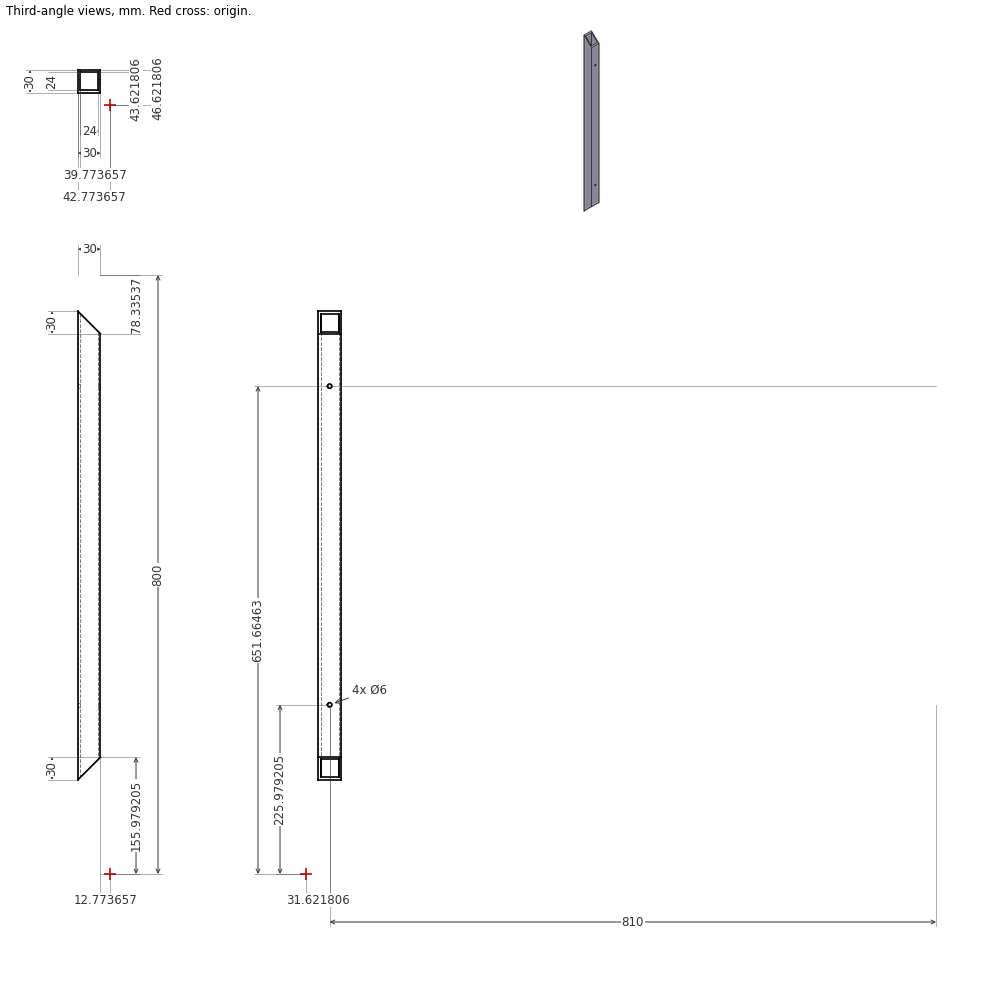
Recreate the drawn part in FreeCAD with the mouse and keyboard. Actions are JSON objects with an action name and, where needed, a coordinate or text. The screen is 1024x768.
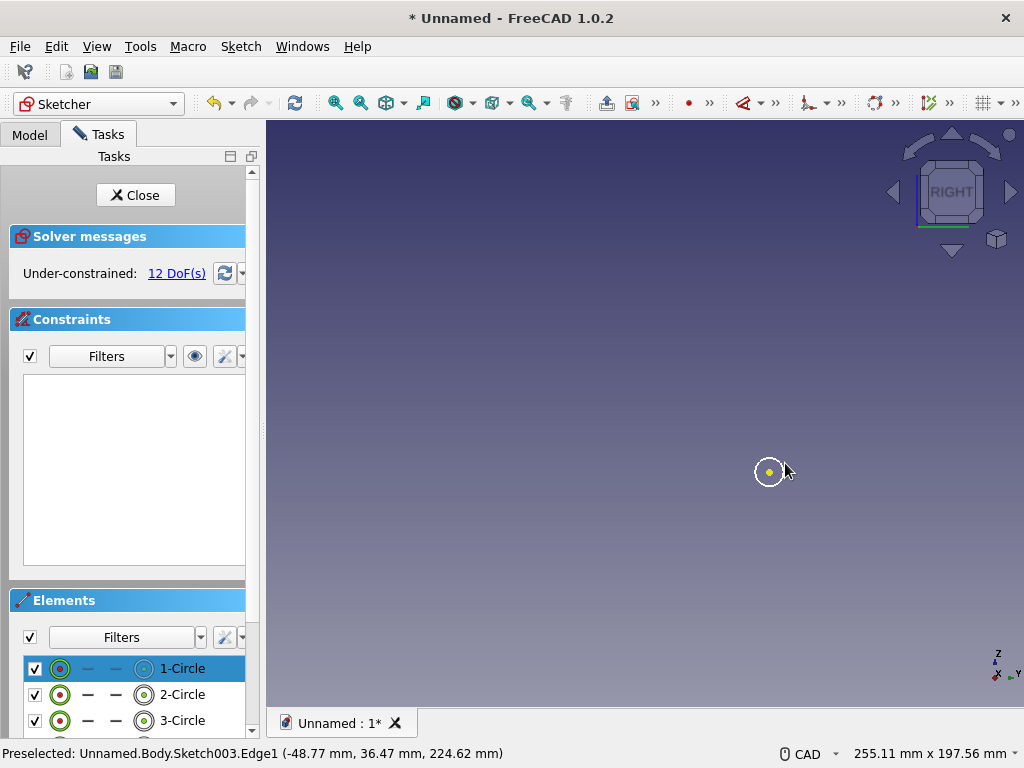
{"action": "left_click", "coordinate": [779, 462]}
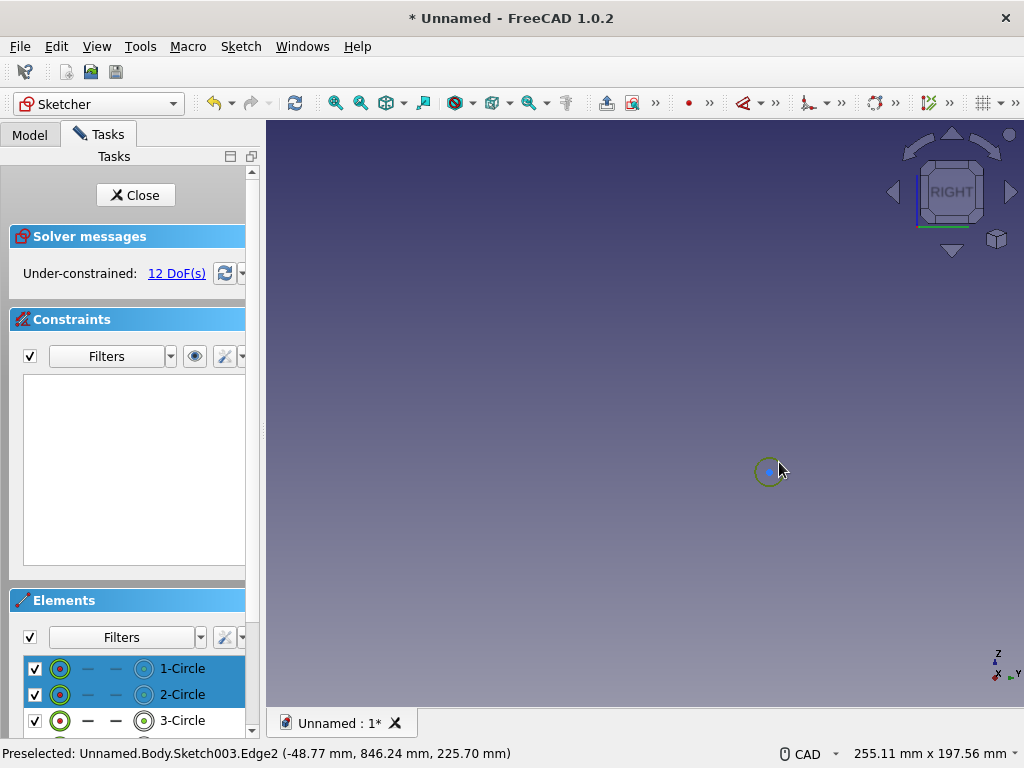
{"action": "scroll", "coordinate": [785, 463], "scroll_direction": "down", "scroll_amount": 9}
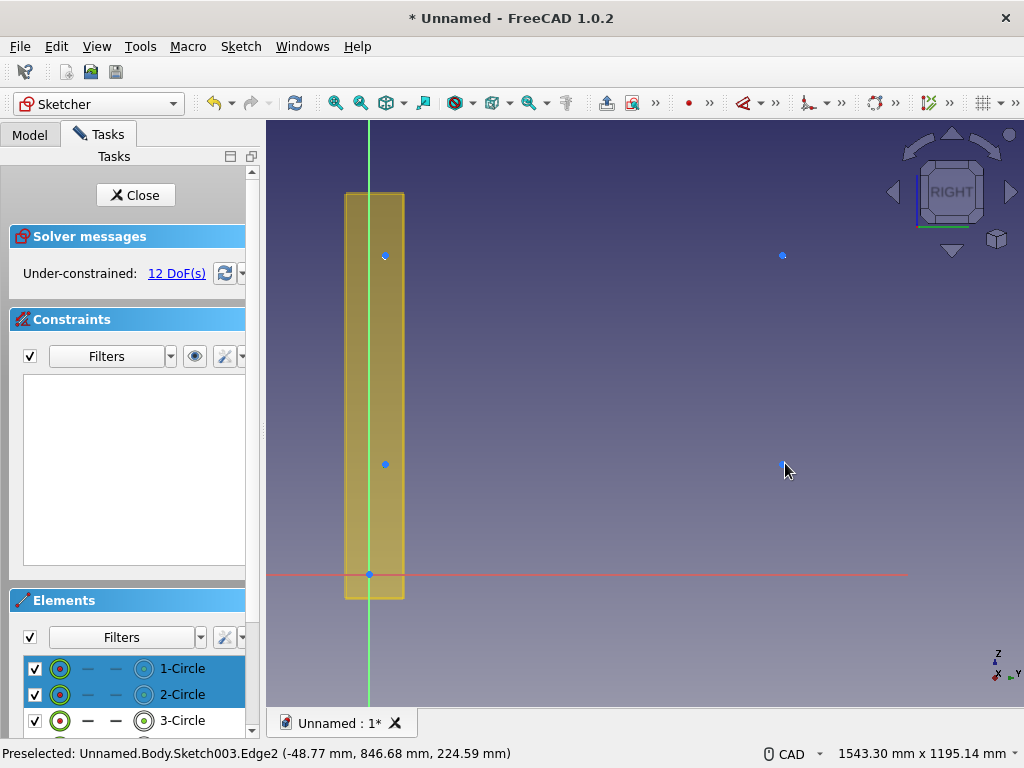
{"action": "scroll", "coordinate": [785, 254], "scroll_direction": "up", "scroll_amount": 9}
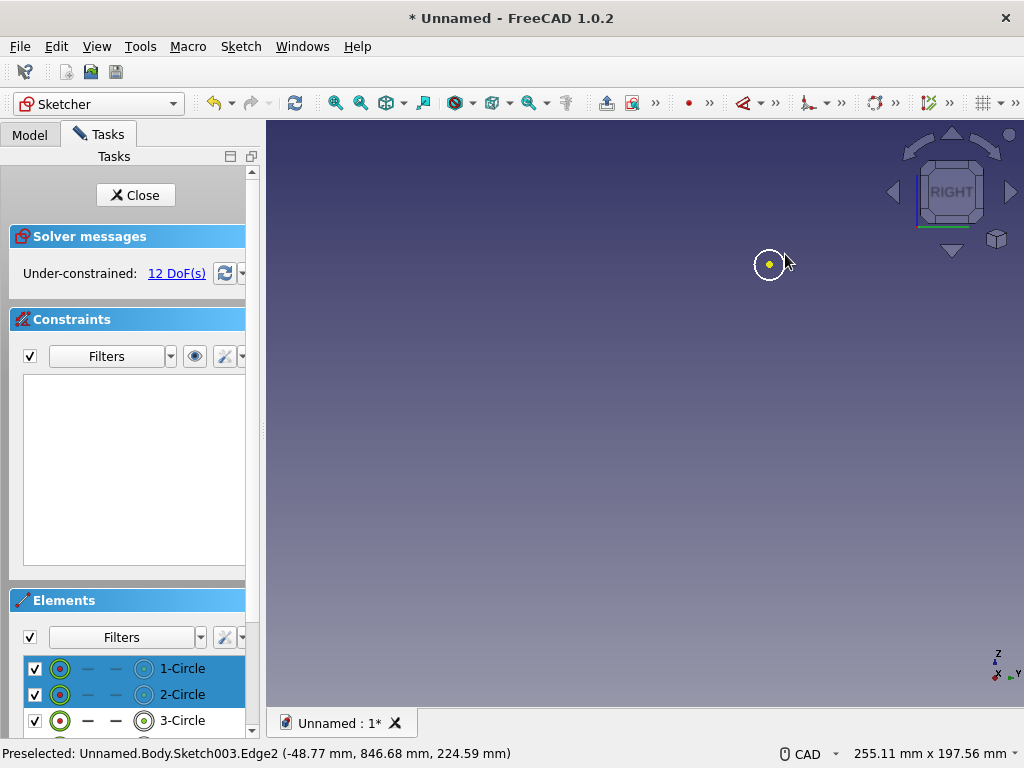
{"action": "left_click", "coordinate": [780, 254]}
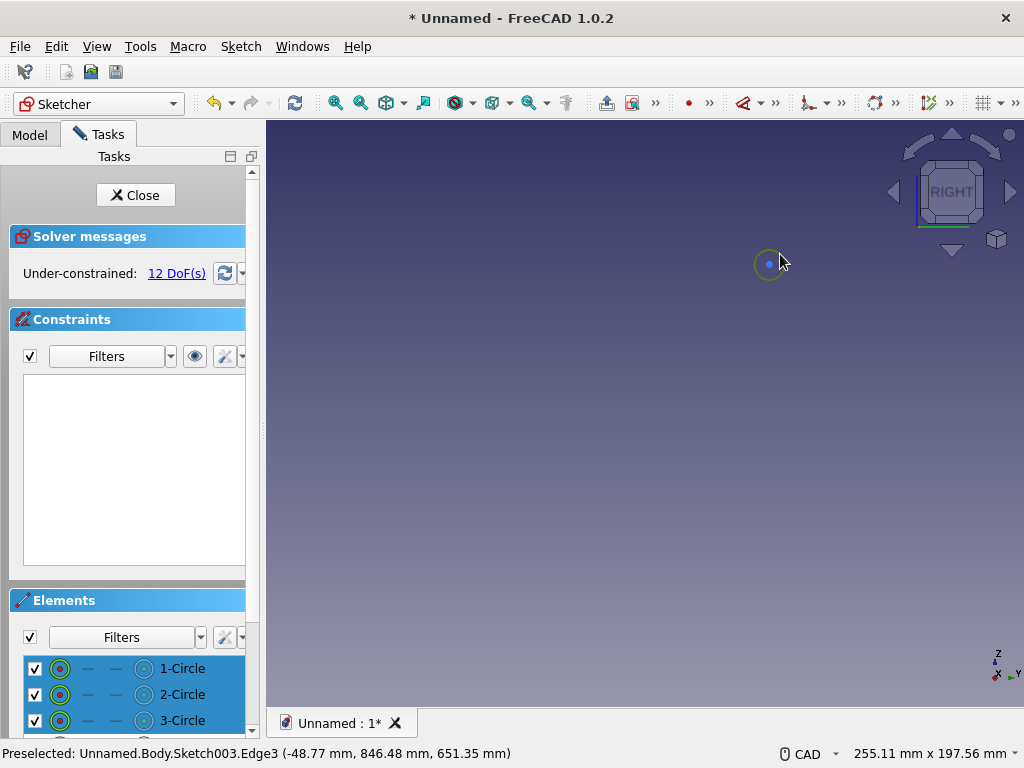
{"action": "scroll", "coordinate": [785, 254], "scroll_direction": "down", "scroll_amount": 9}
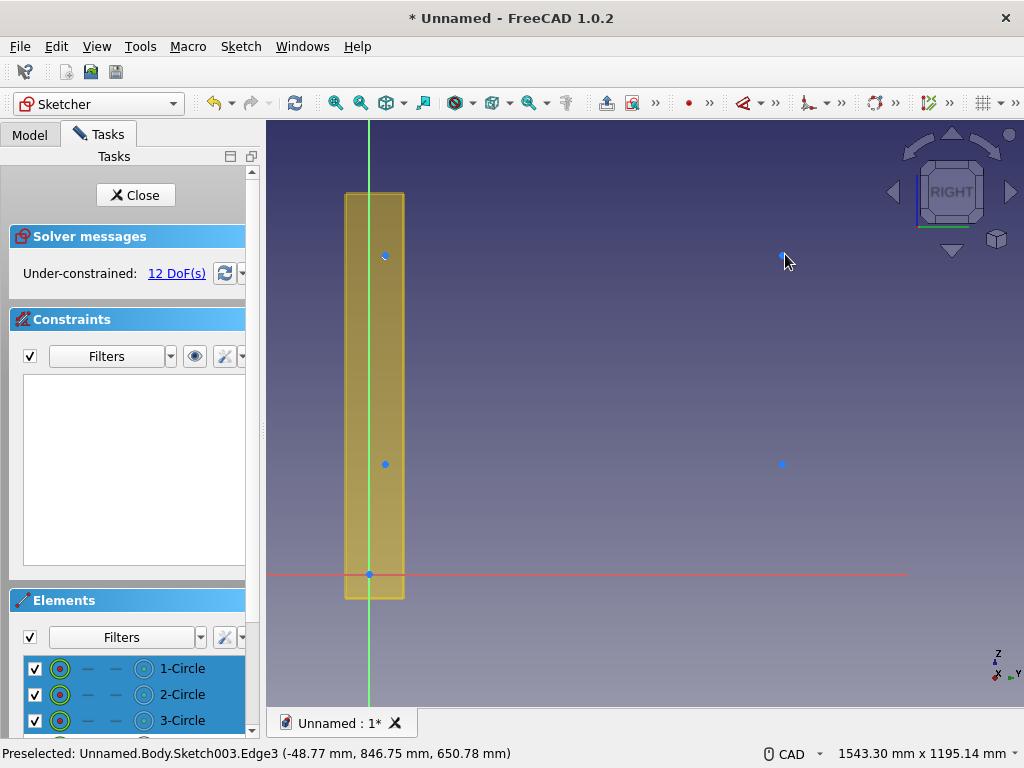
{"action": "scroll", "coordinate": [387, 254], "scroll_direction": "up", "scroll_amount": 9}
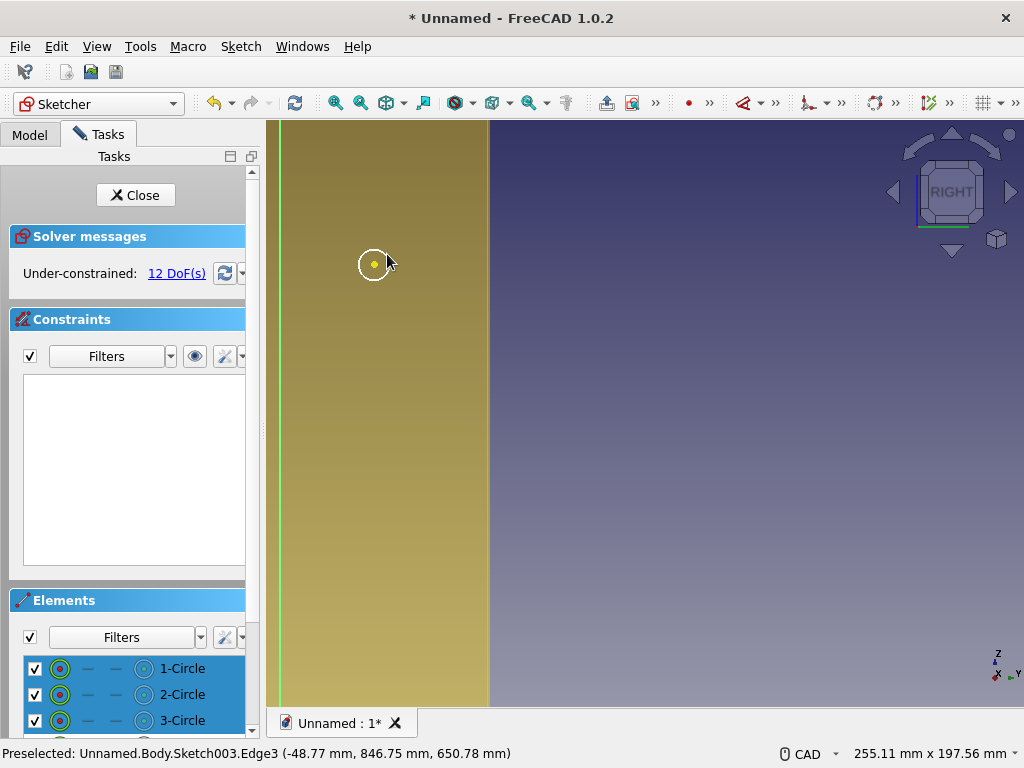
{"action": "left_click", "coordinate": [385, 254]}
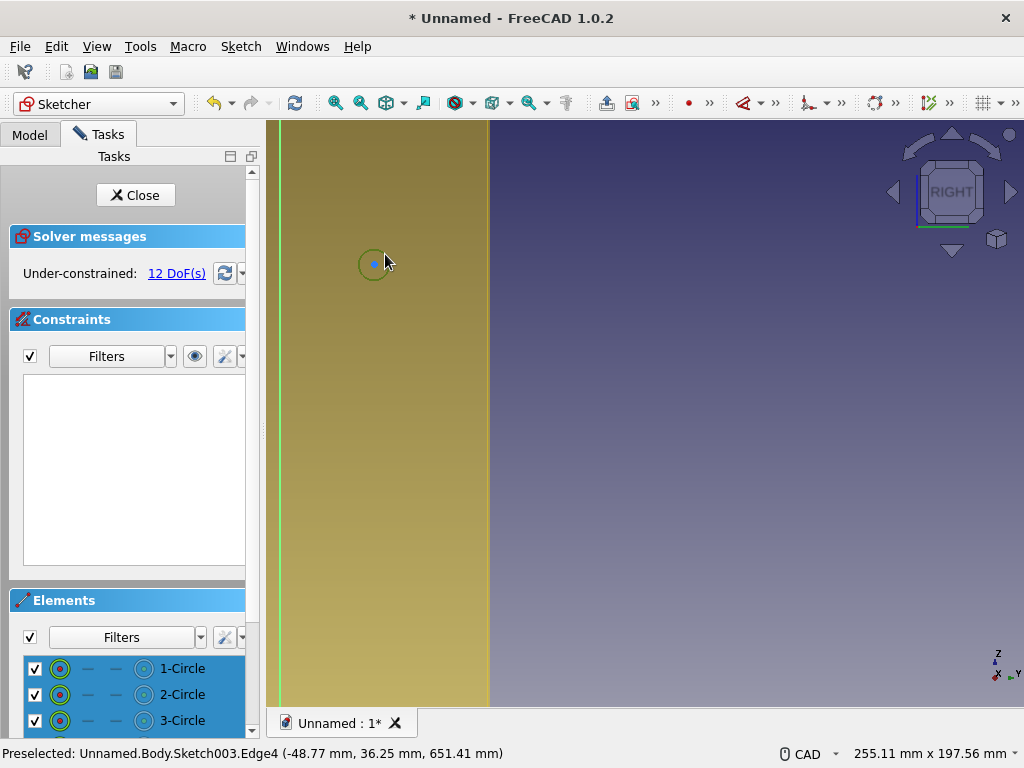
{"action": "key", "text": "e"}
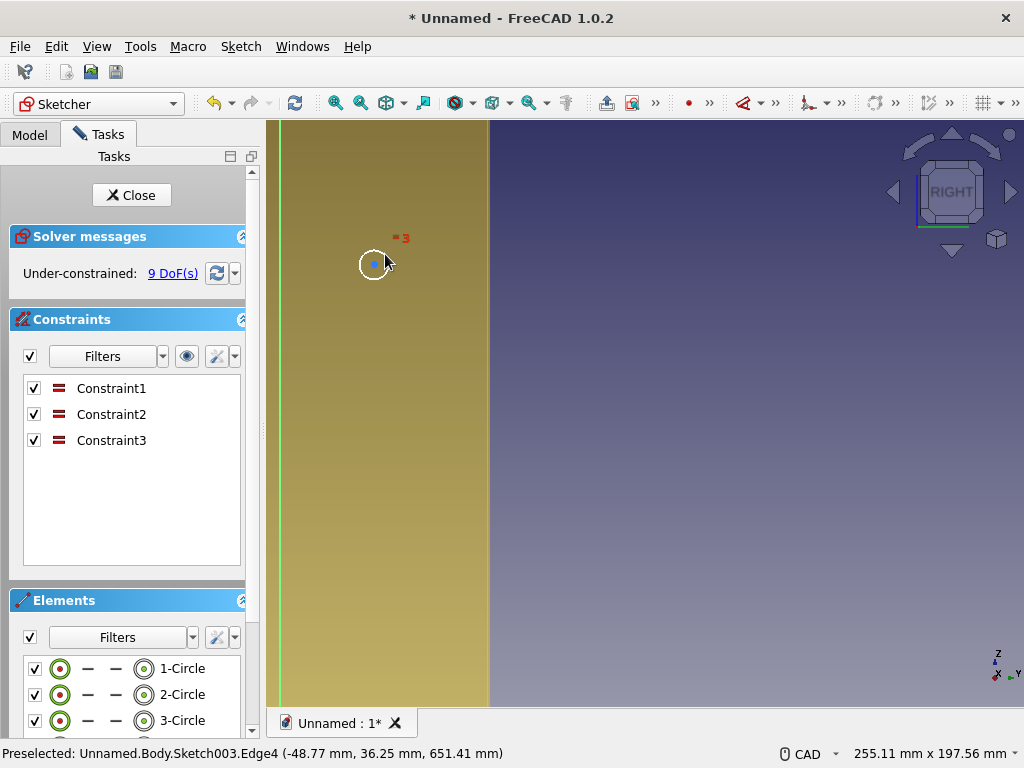
{"action": "scroll", "coordinate": [387, 254], "scroll_direction": "down", "scroll_amount": 9}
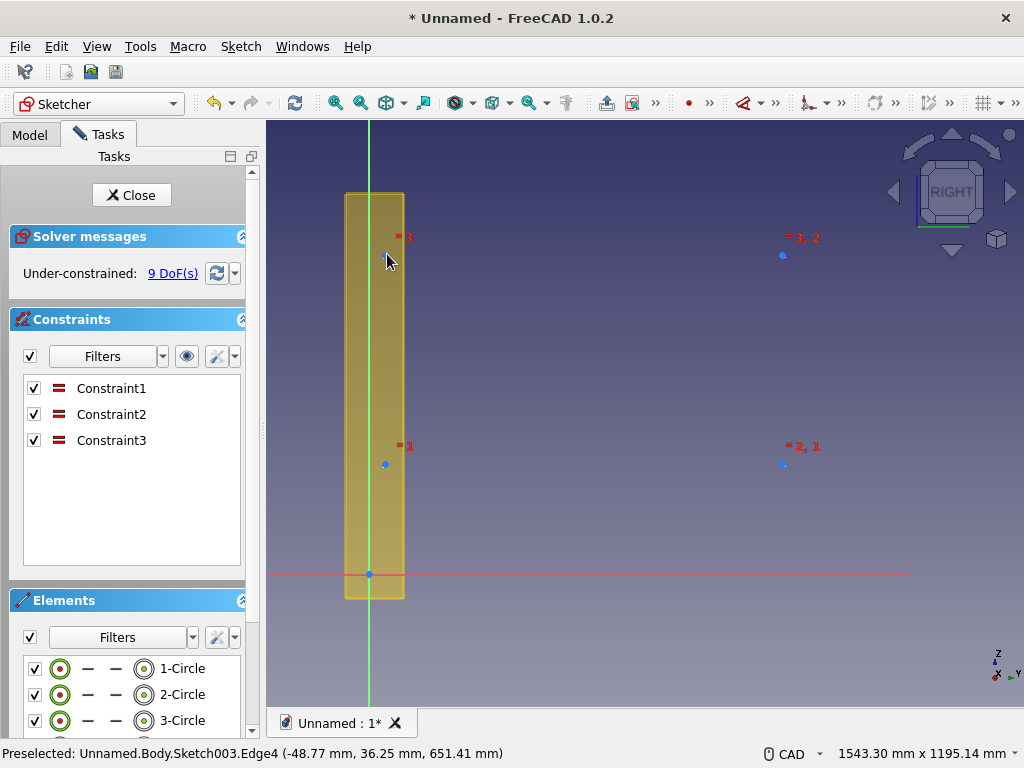
{"action": "left_click", "coordinate": [385, 465]}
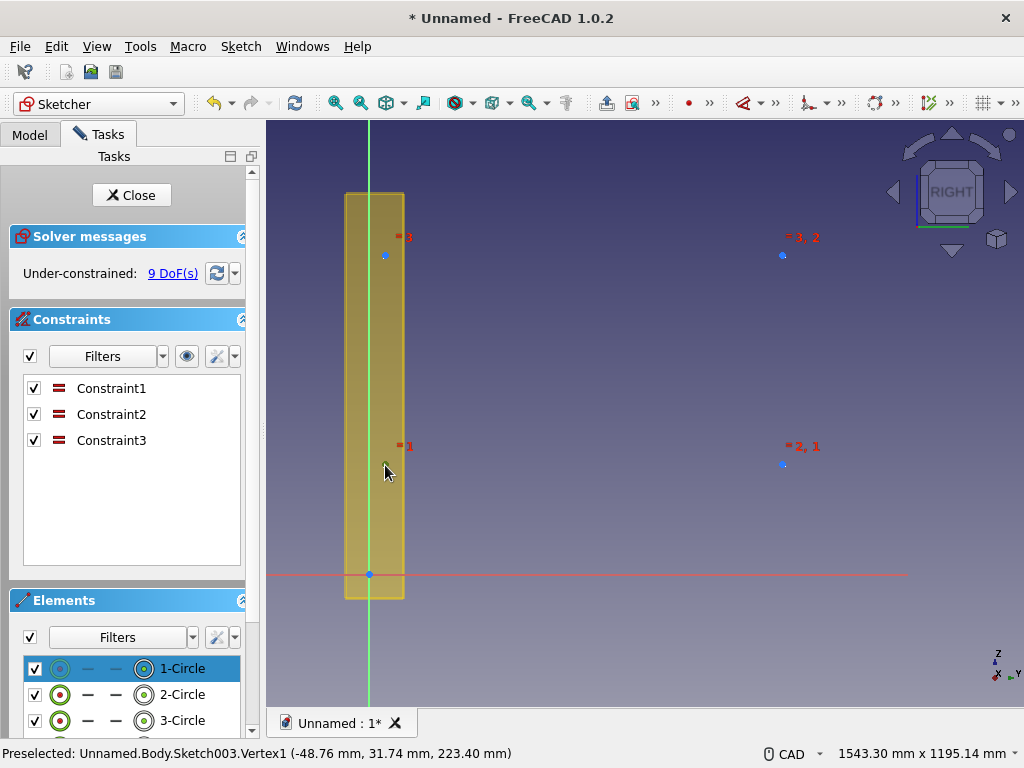
{"action": "left_click", "coordinate": [783, 465]}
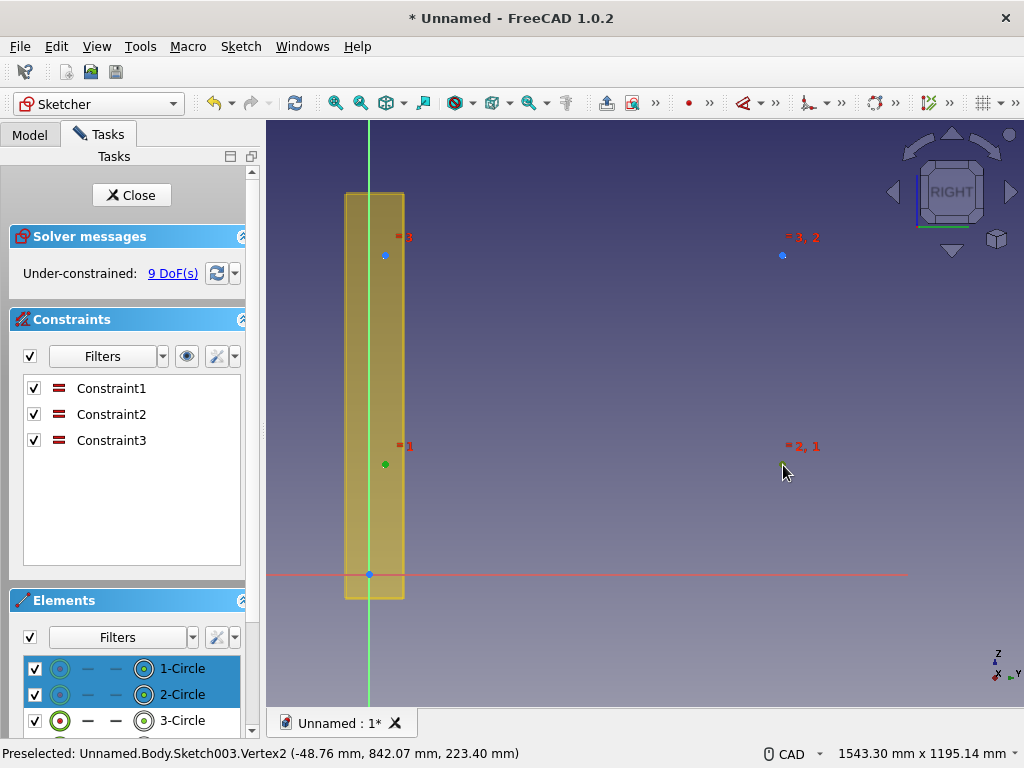
{"action": "key", "text": "h"}